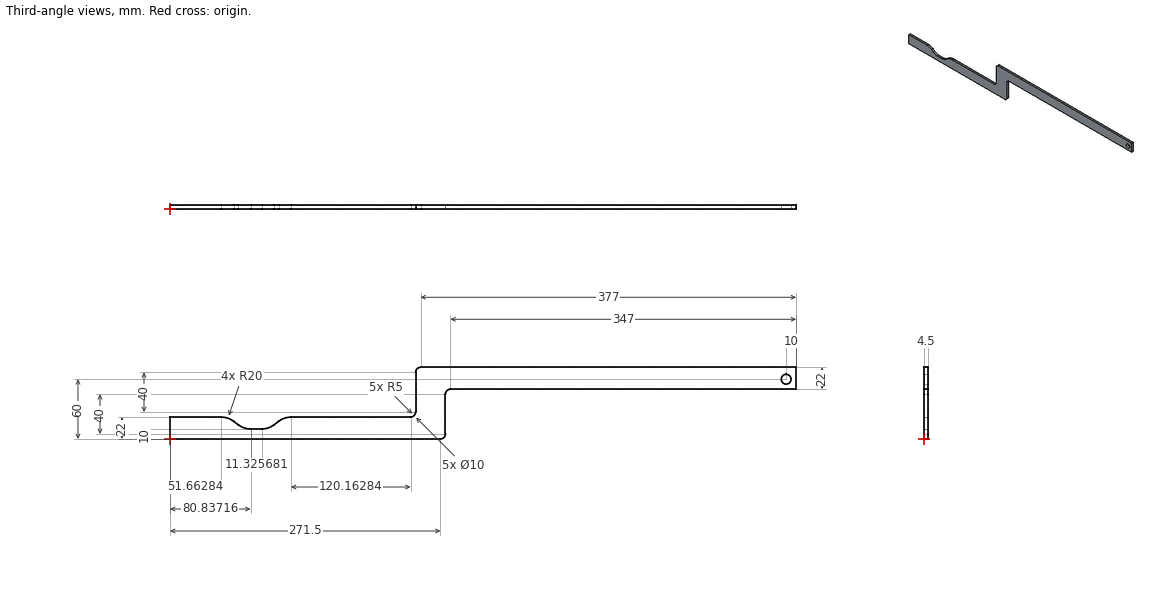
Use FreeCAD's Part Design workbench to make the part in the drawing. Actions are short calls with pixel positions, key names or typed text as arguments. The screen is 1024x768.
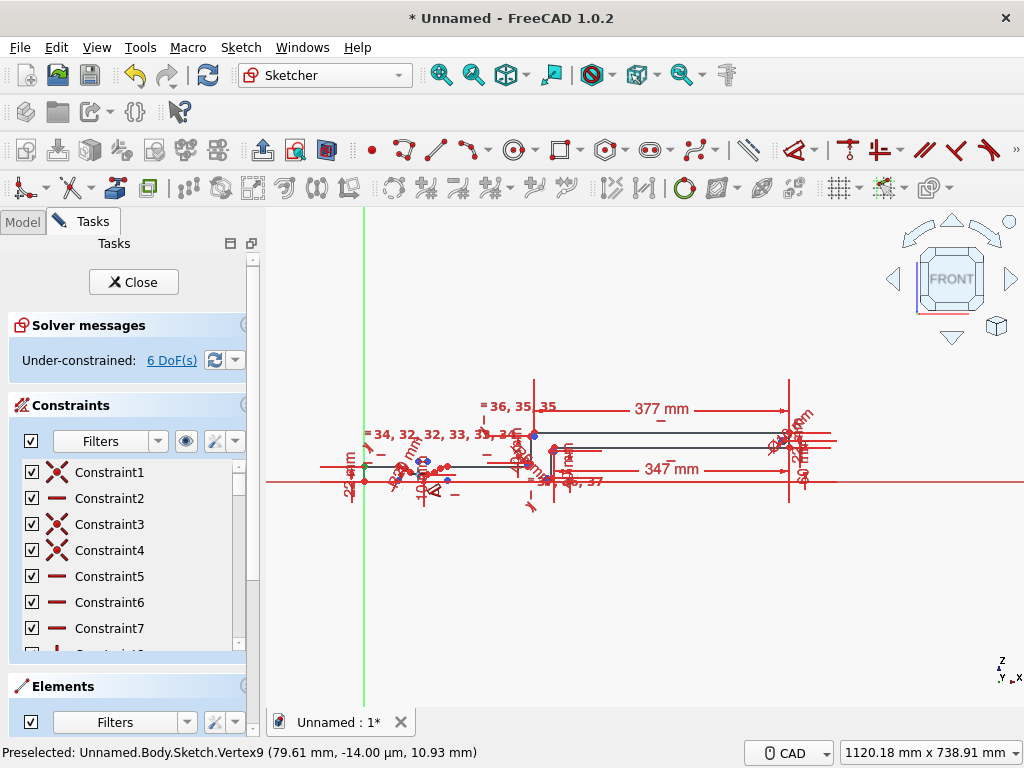
scroll(789, 448, up, 9)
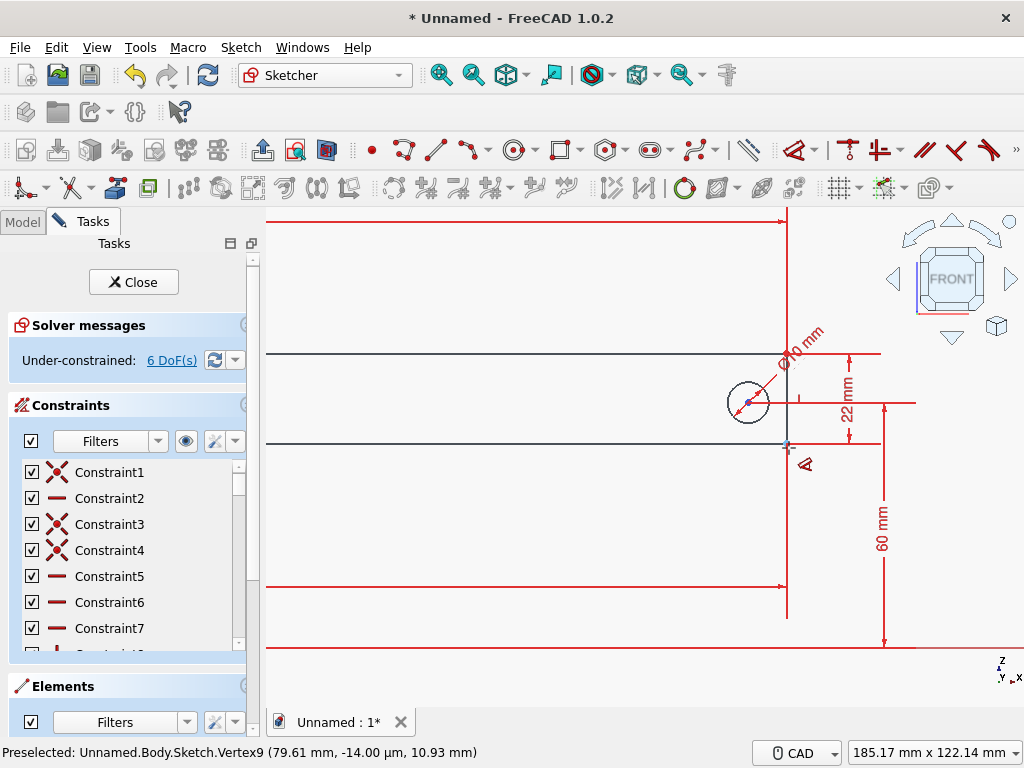
click(787, 444)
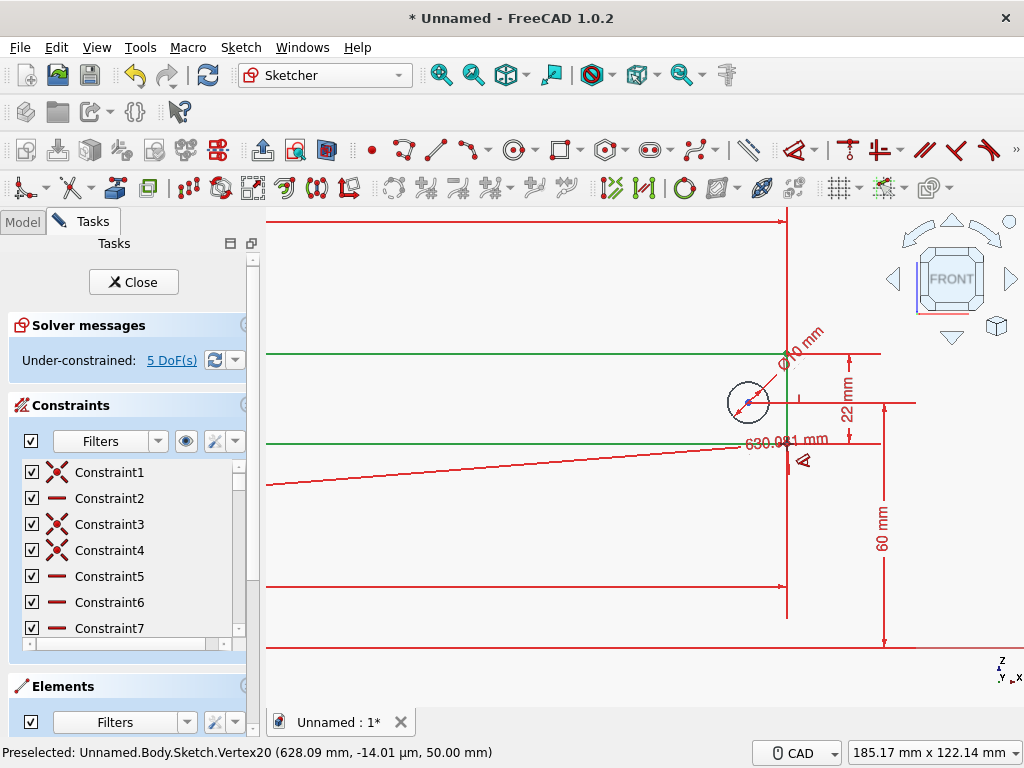
click(748, 403)
click(768, 478)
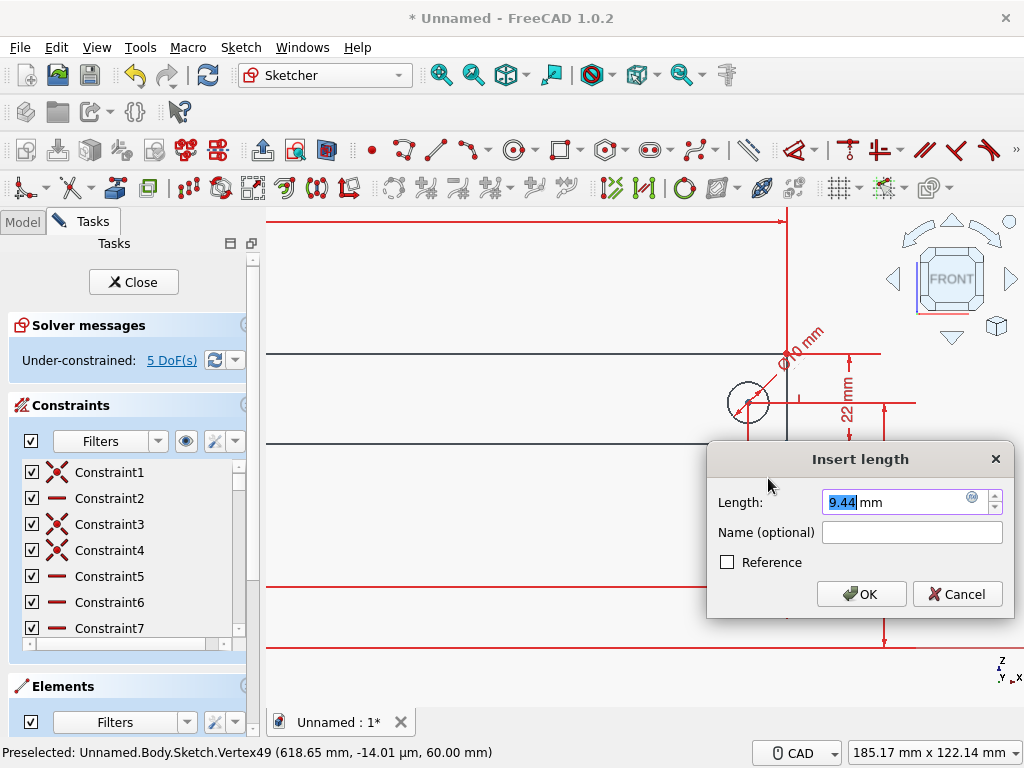
text(10)
key(Return)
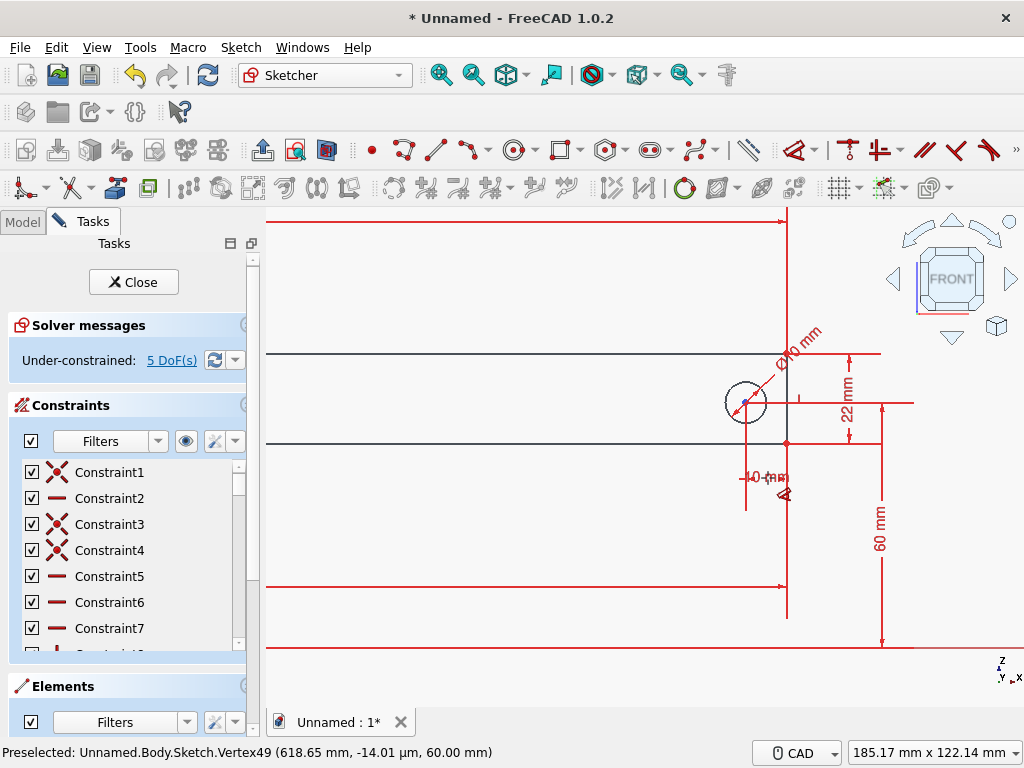
scroll(789, 448, down, 9)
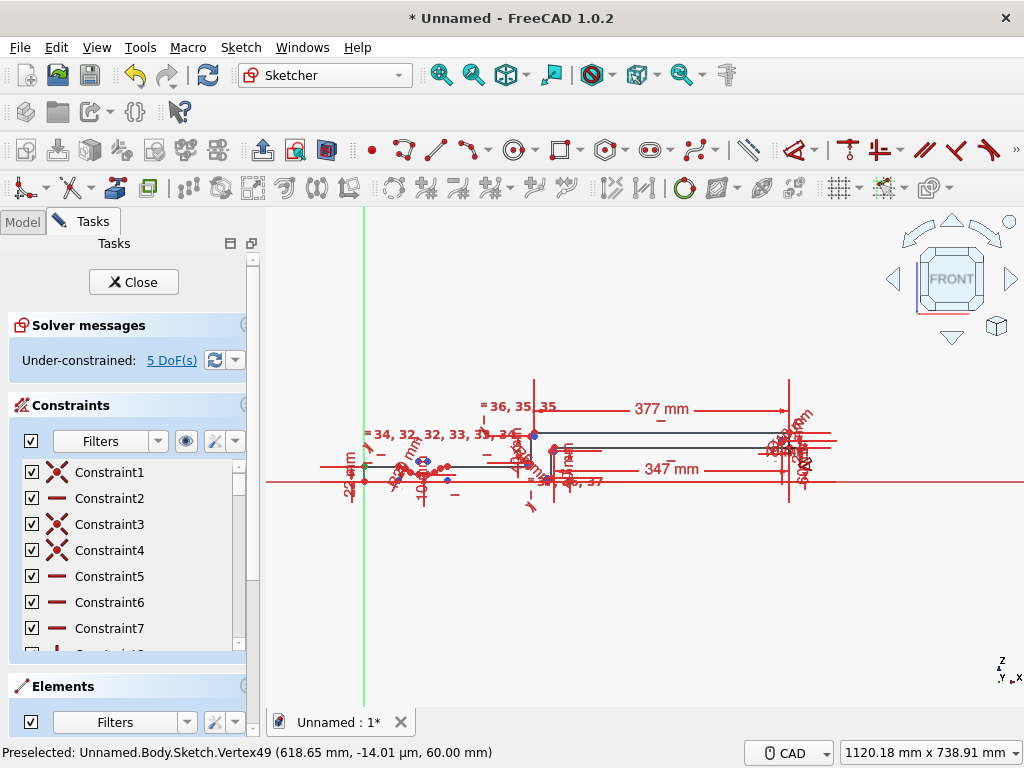
click(493, 482)
click(456, 516)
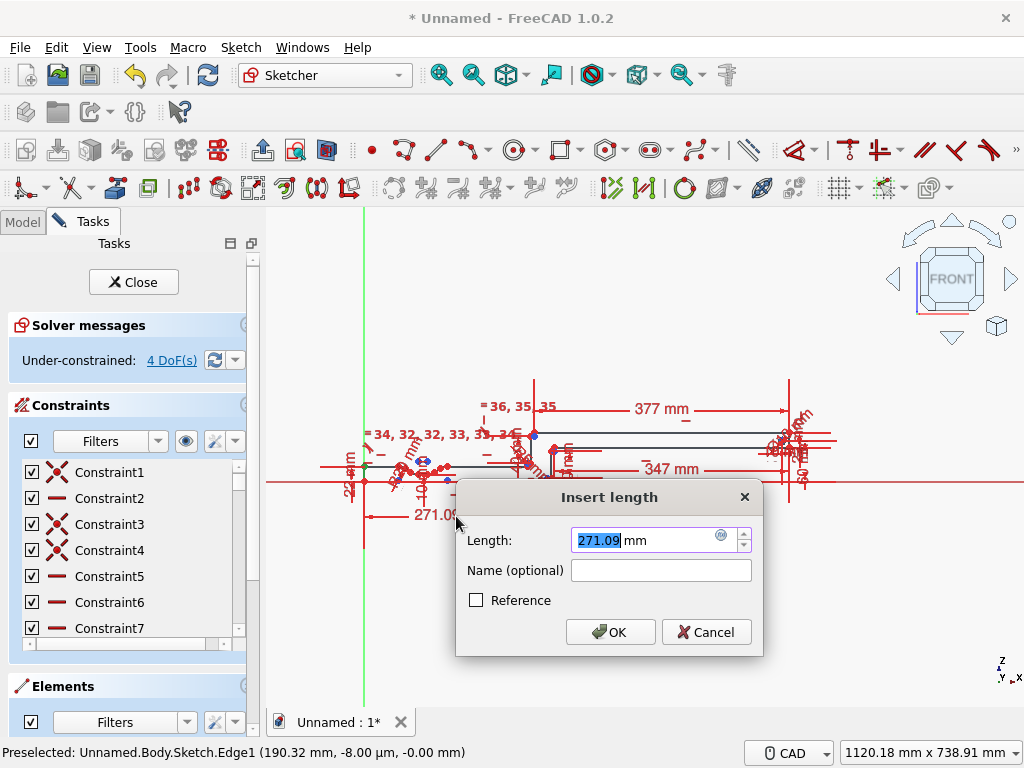
text(271.5)
key(Return)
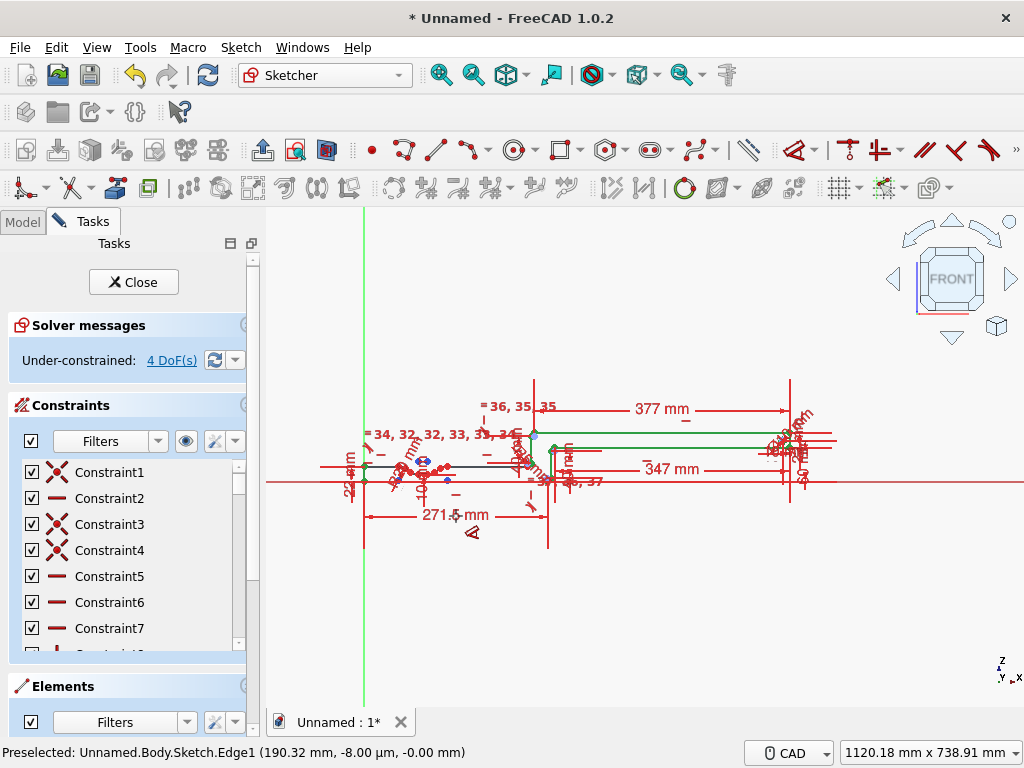
scroll(374, 467, up, 2)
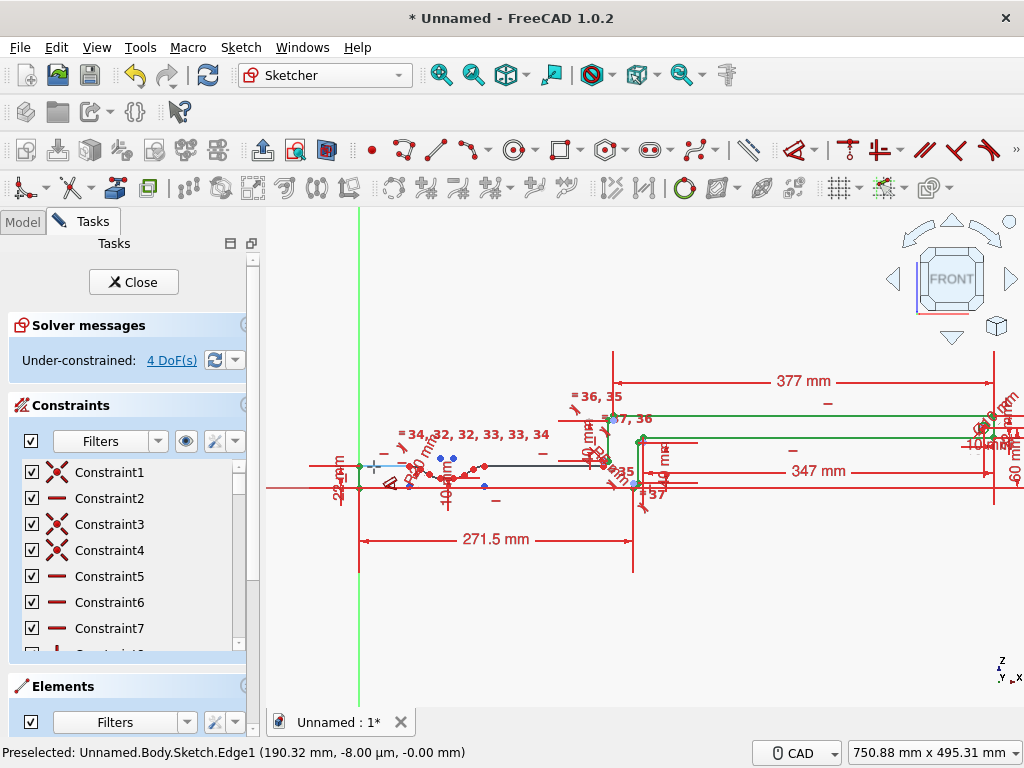
click(374, 466)
click(385, 432)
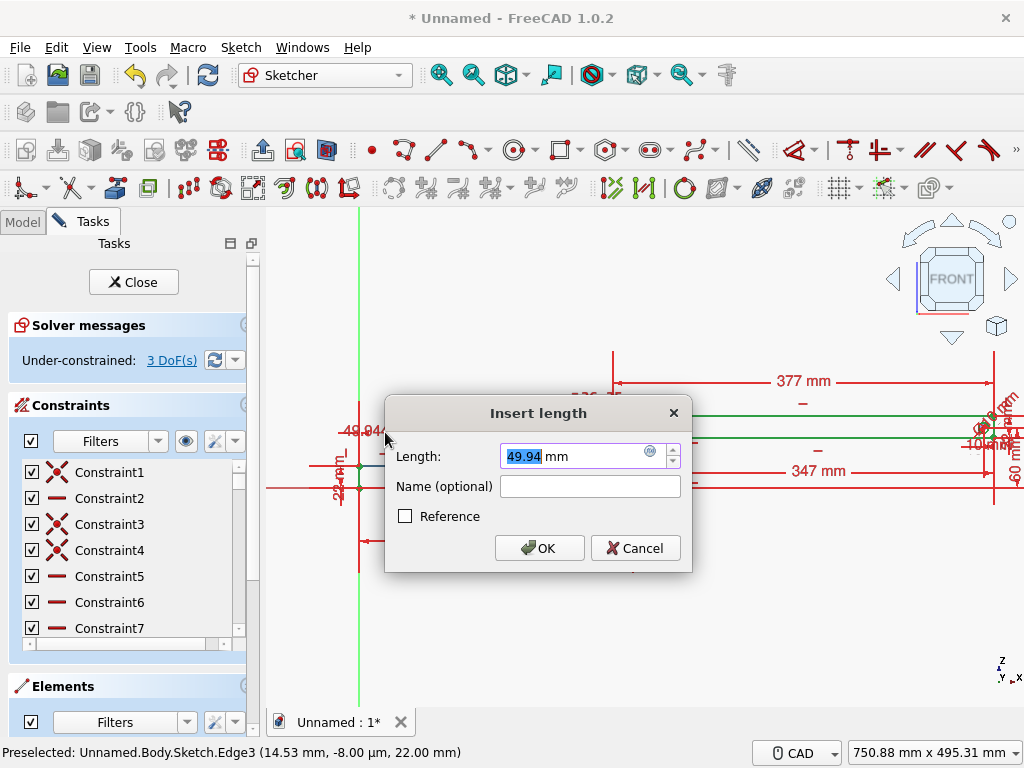
text(51.66284)
key(Return)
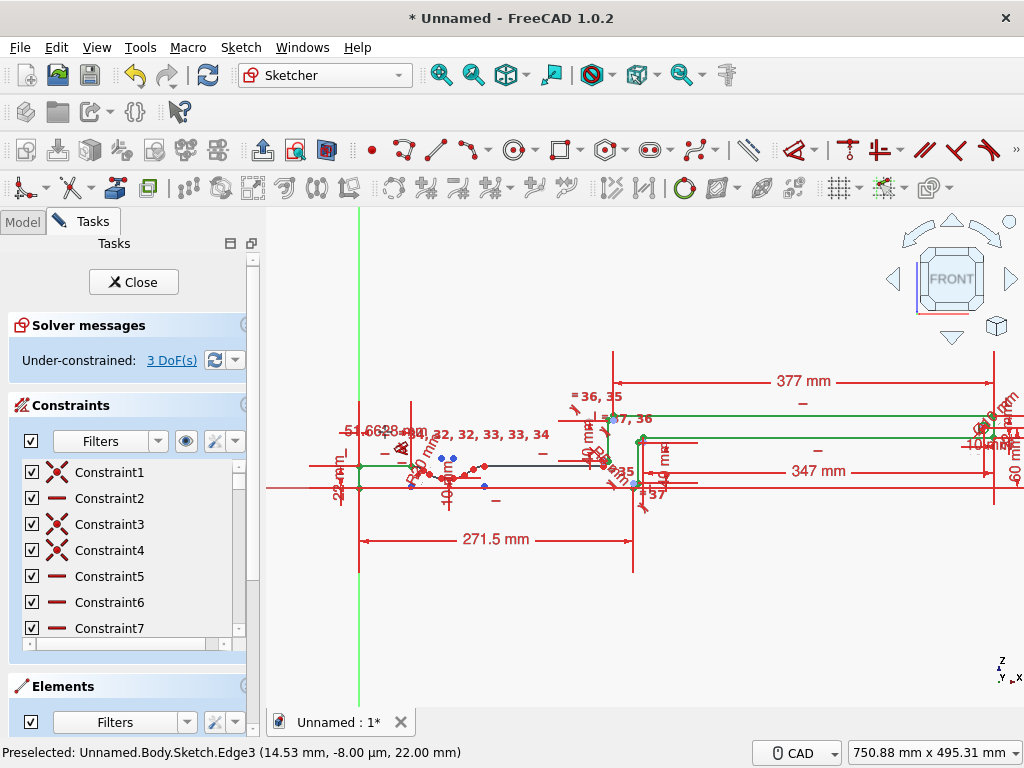
scroll(447, 478, up, 7)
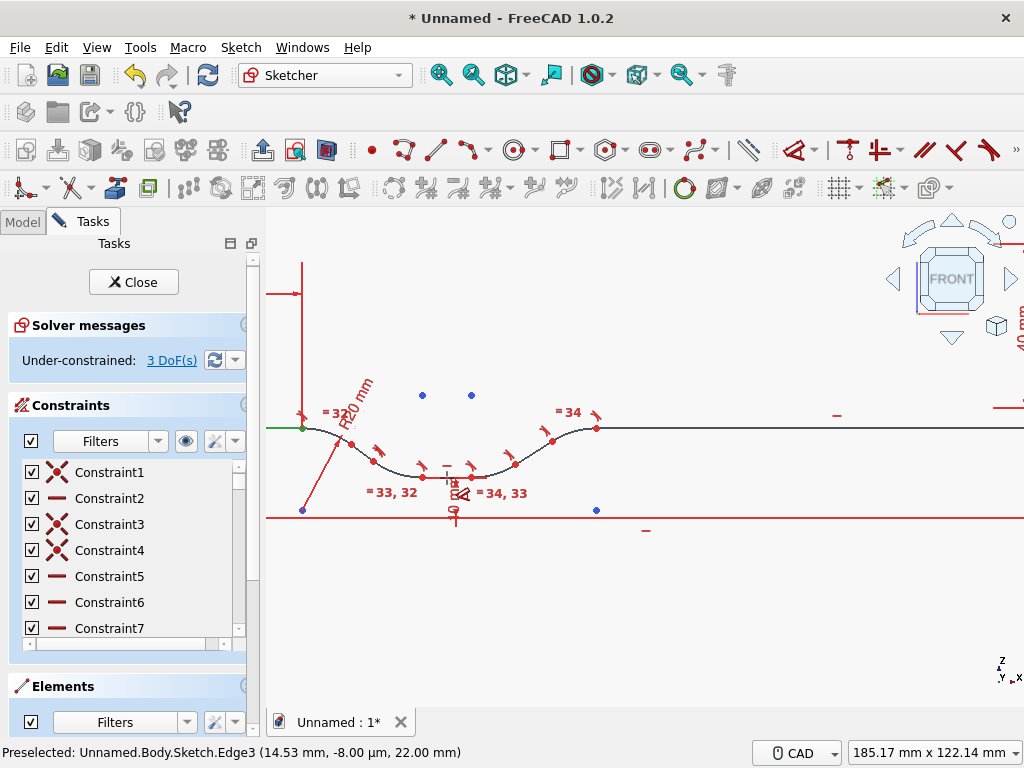
click(447, 478)
click(447, 444)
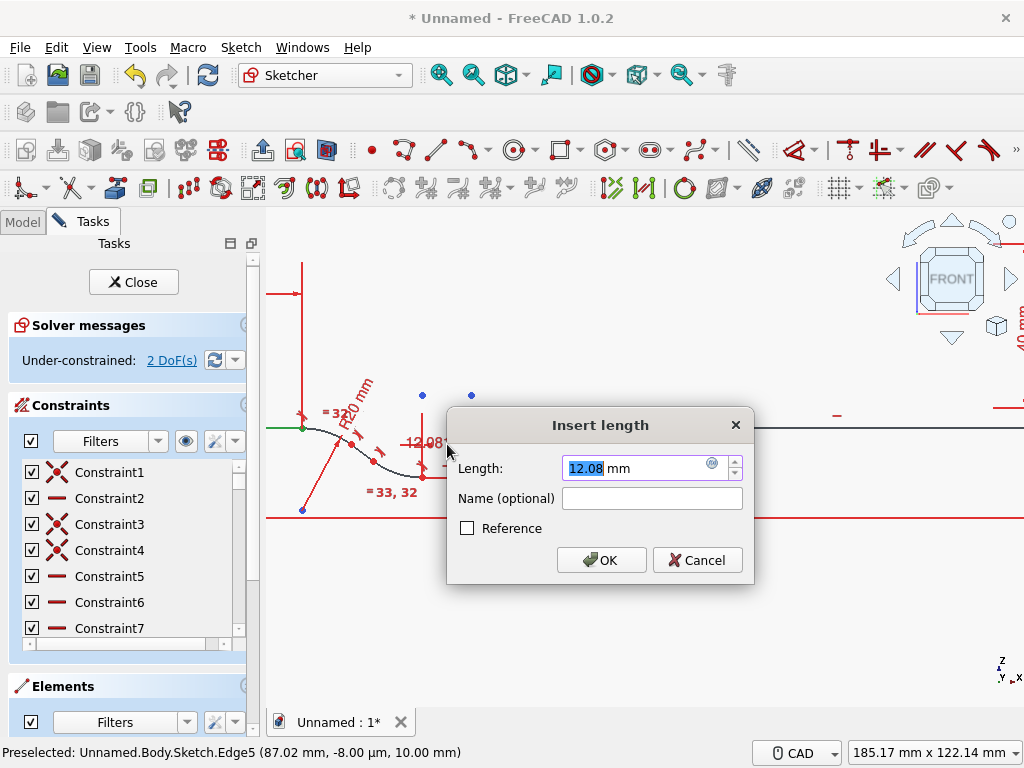
text(11.325681)
key(Return)